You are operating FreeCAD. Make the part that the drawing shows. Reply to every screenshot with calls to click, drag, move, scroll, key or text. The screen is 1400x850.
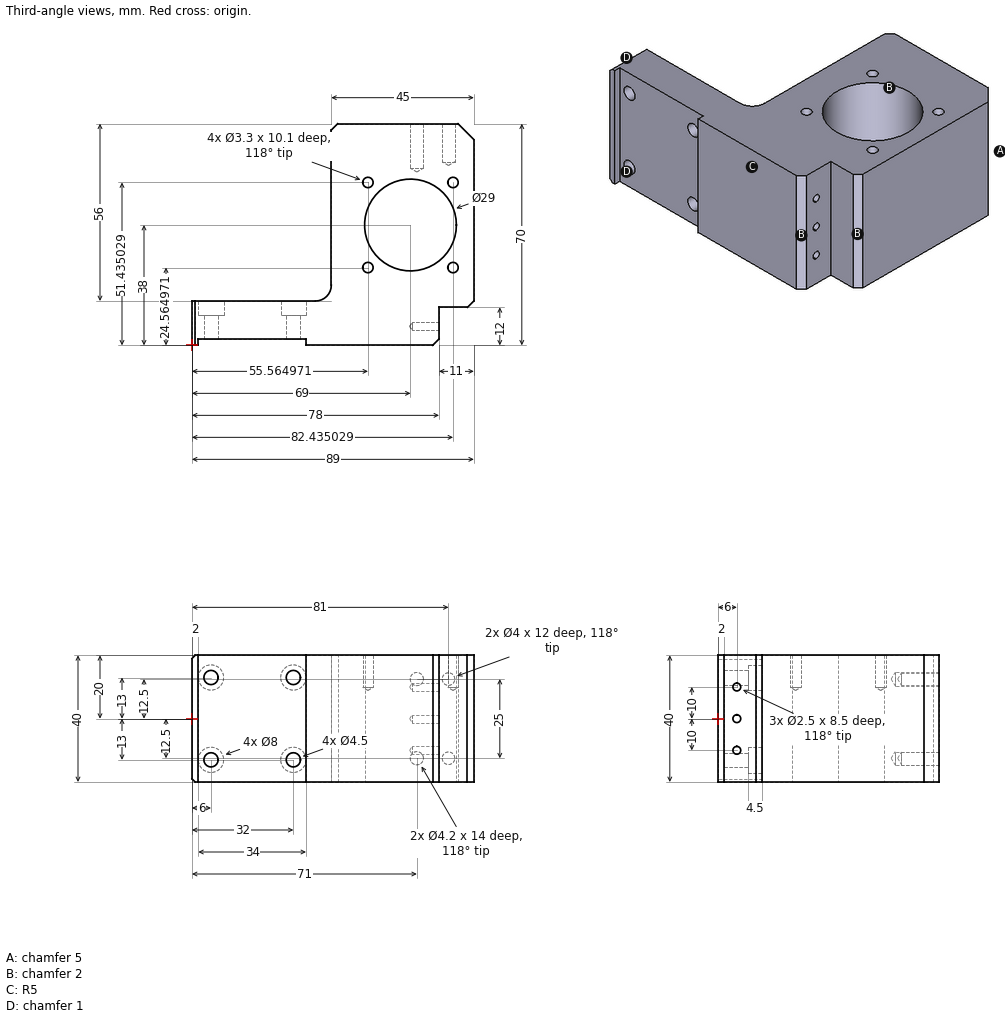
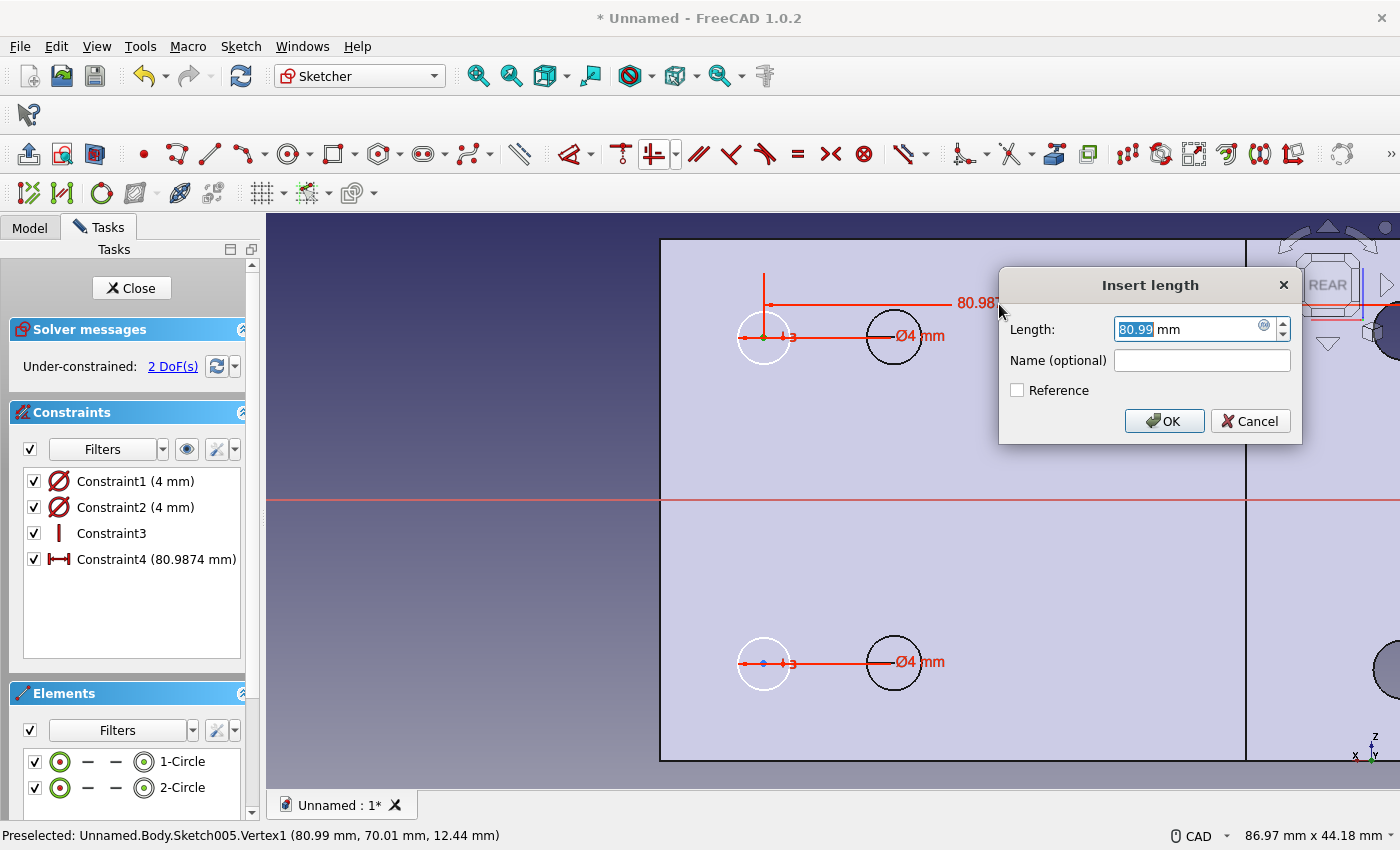
text(81)
key(Return)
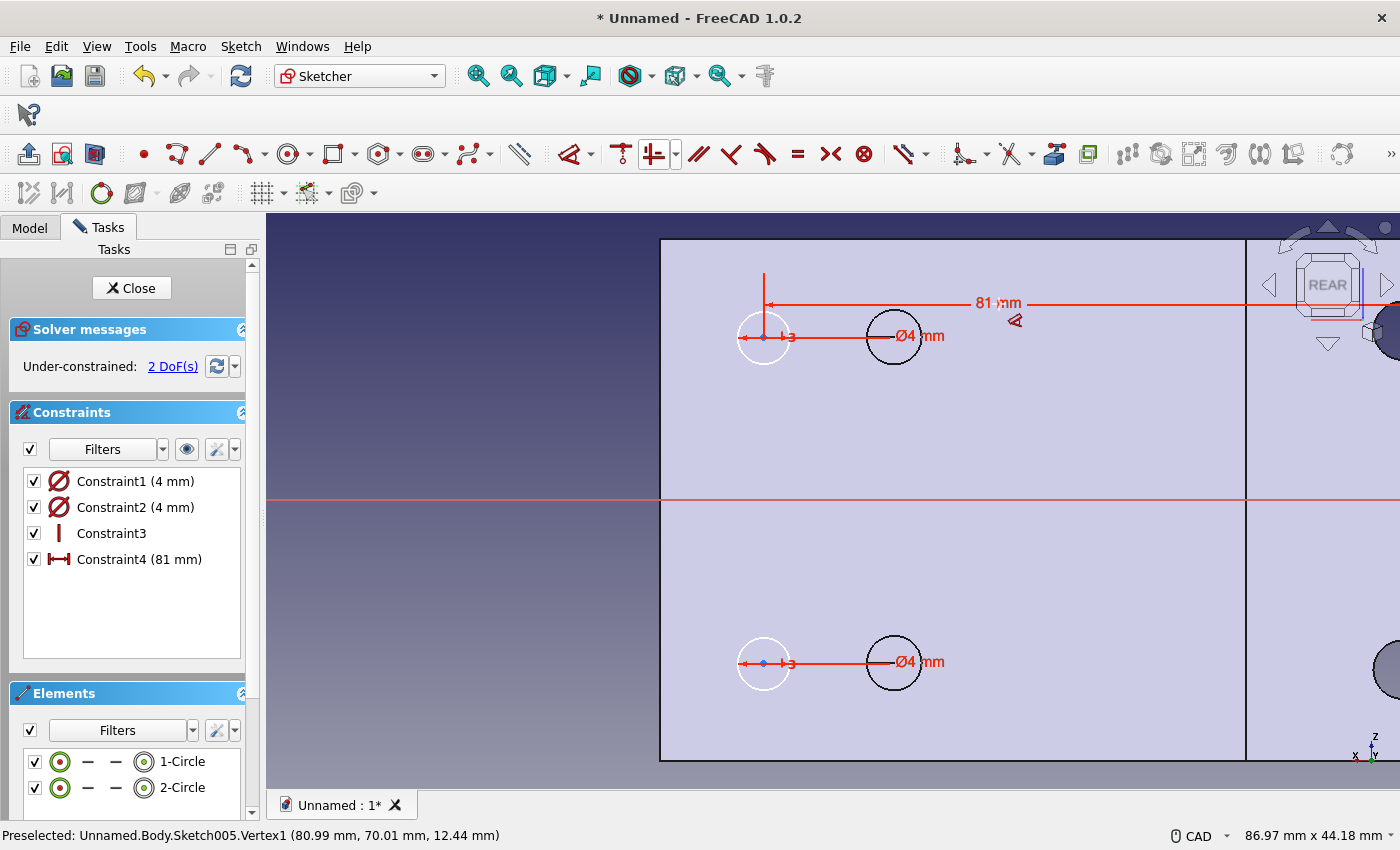
click(764, 338)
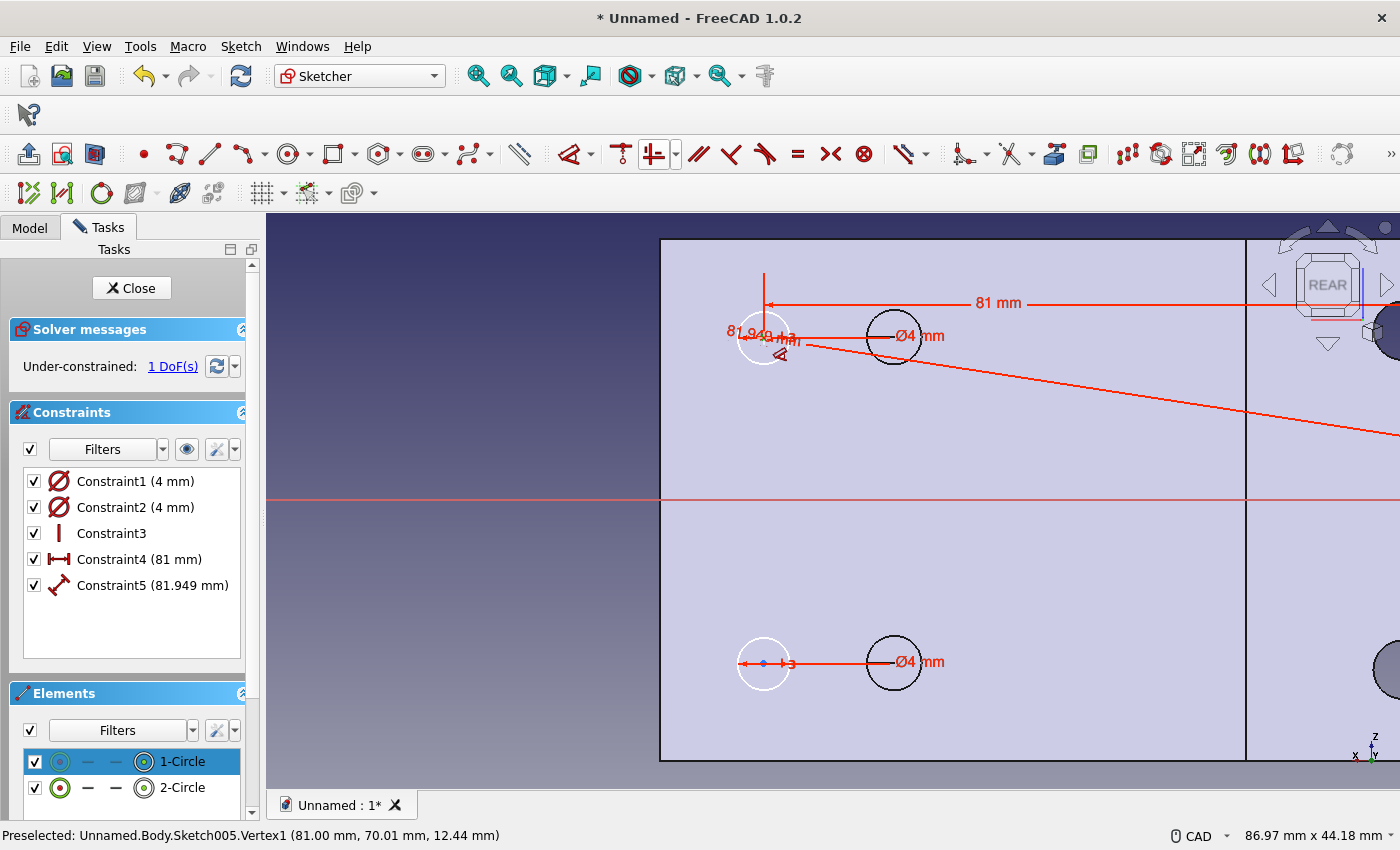
click(764, 664)
click(798, 426)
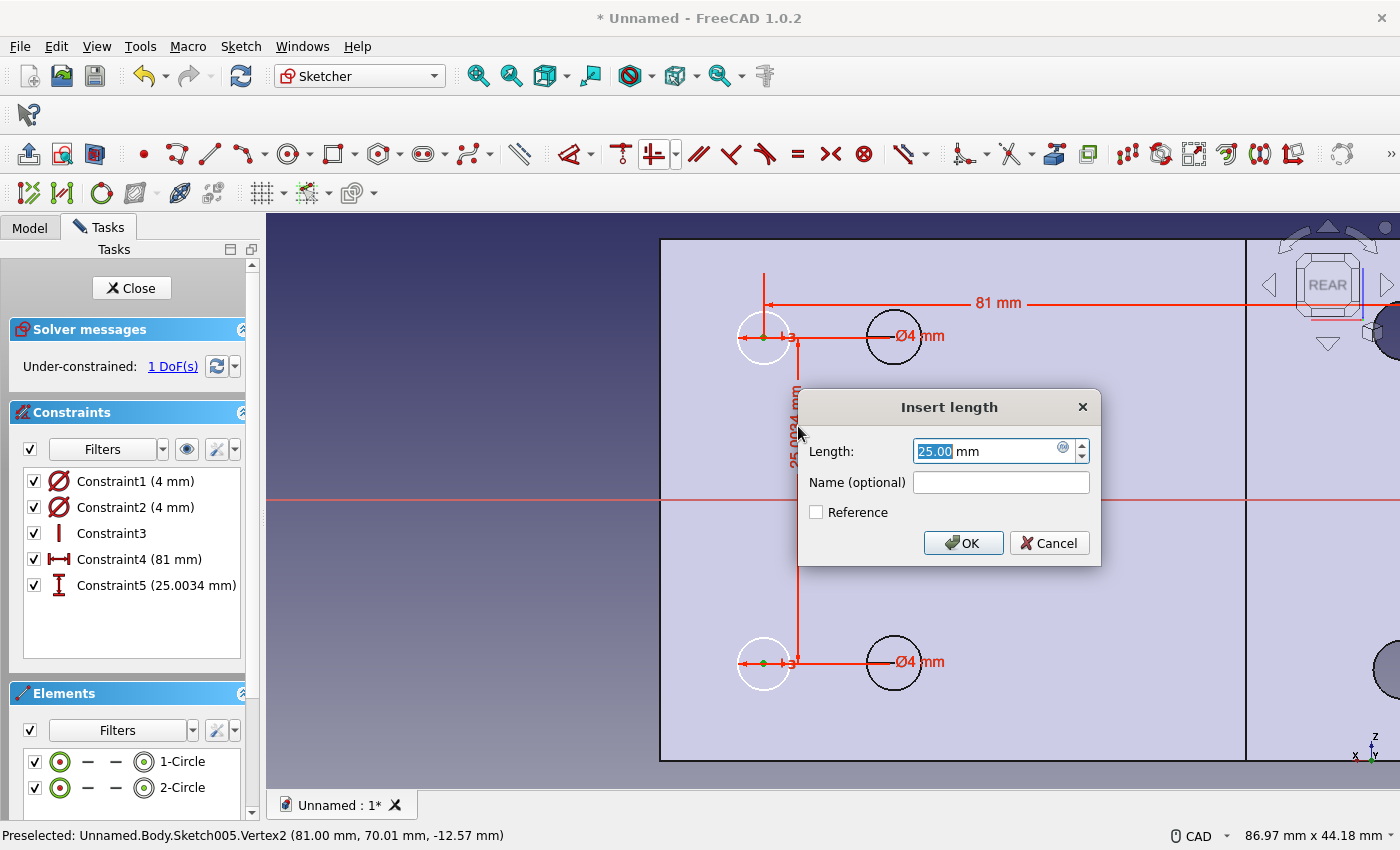
text(25)
key(Return)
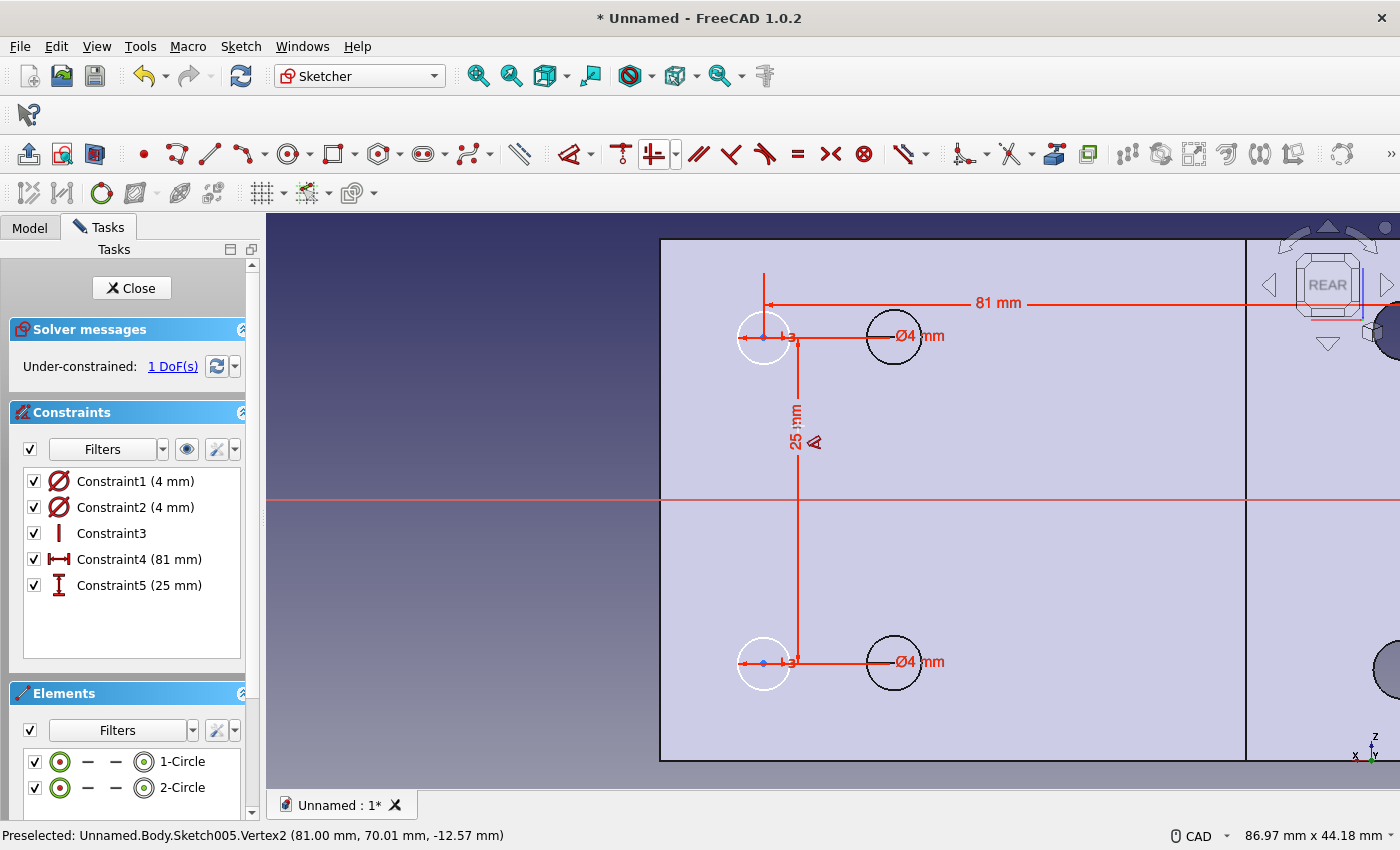
click(764, 338)
click(730, 382)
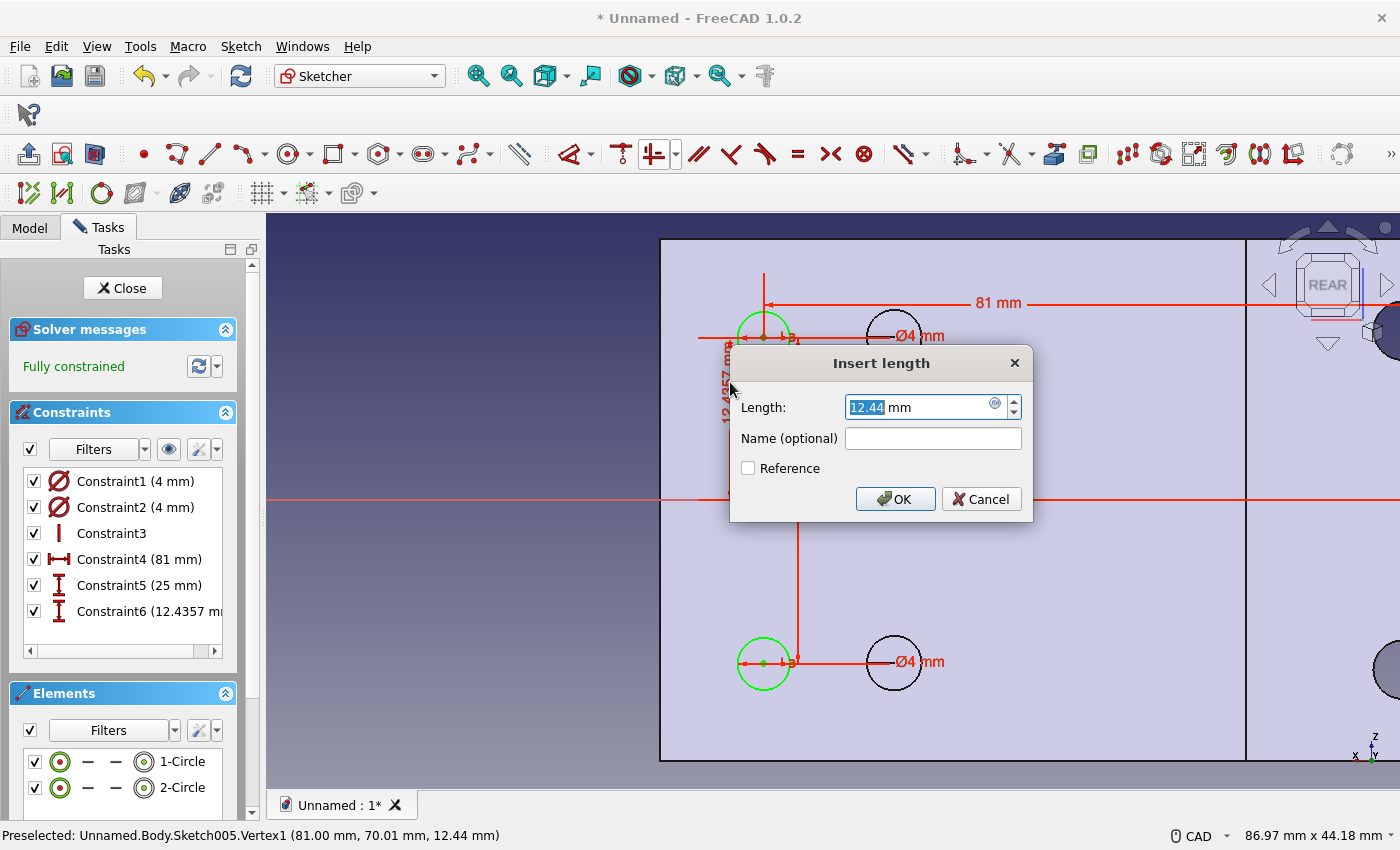
text(12.5)
key(Return)
key(Escape)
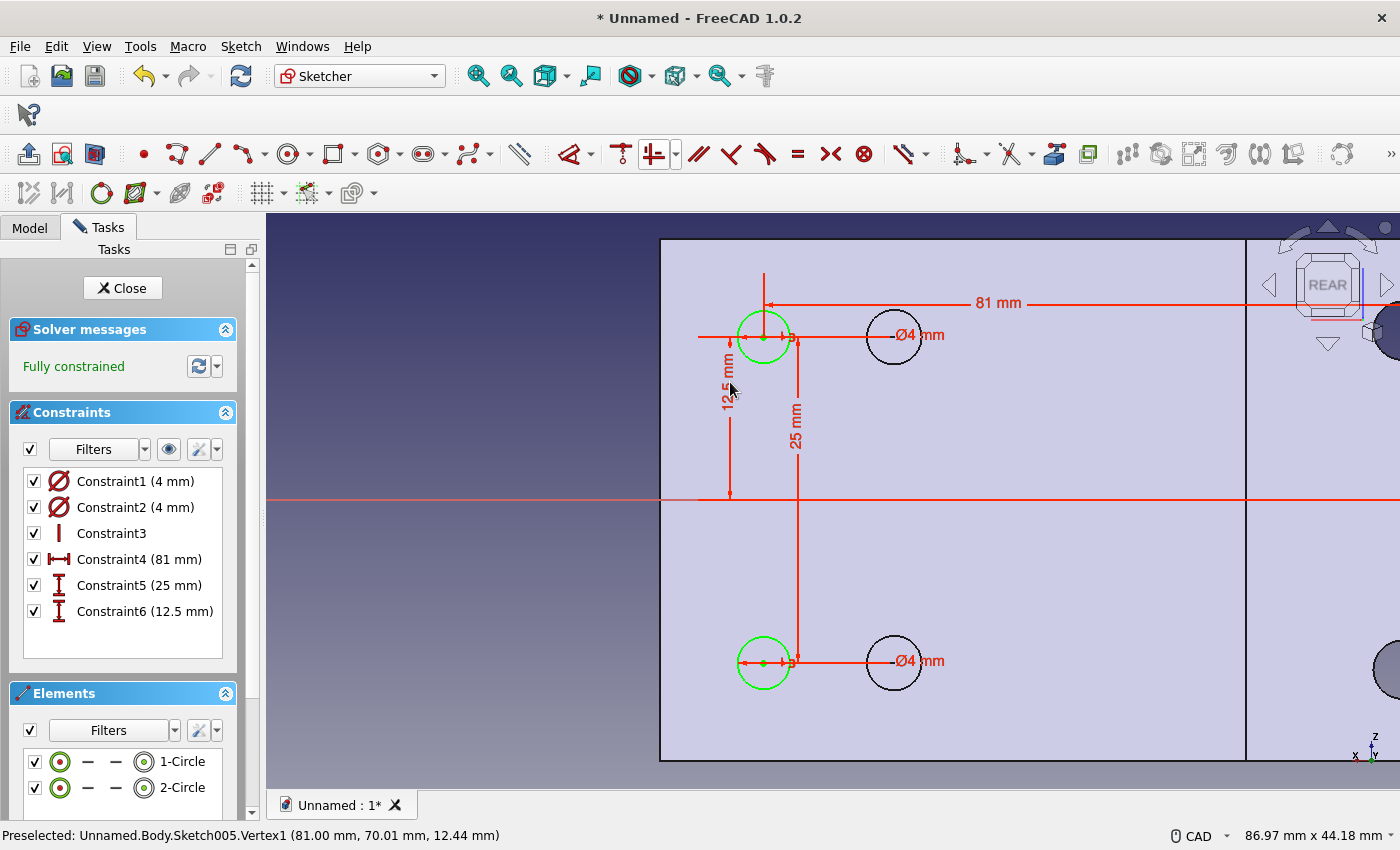
click(123, 288)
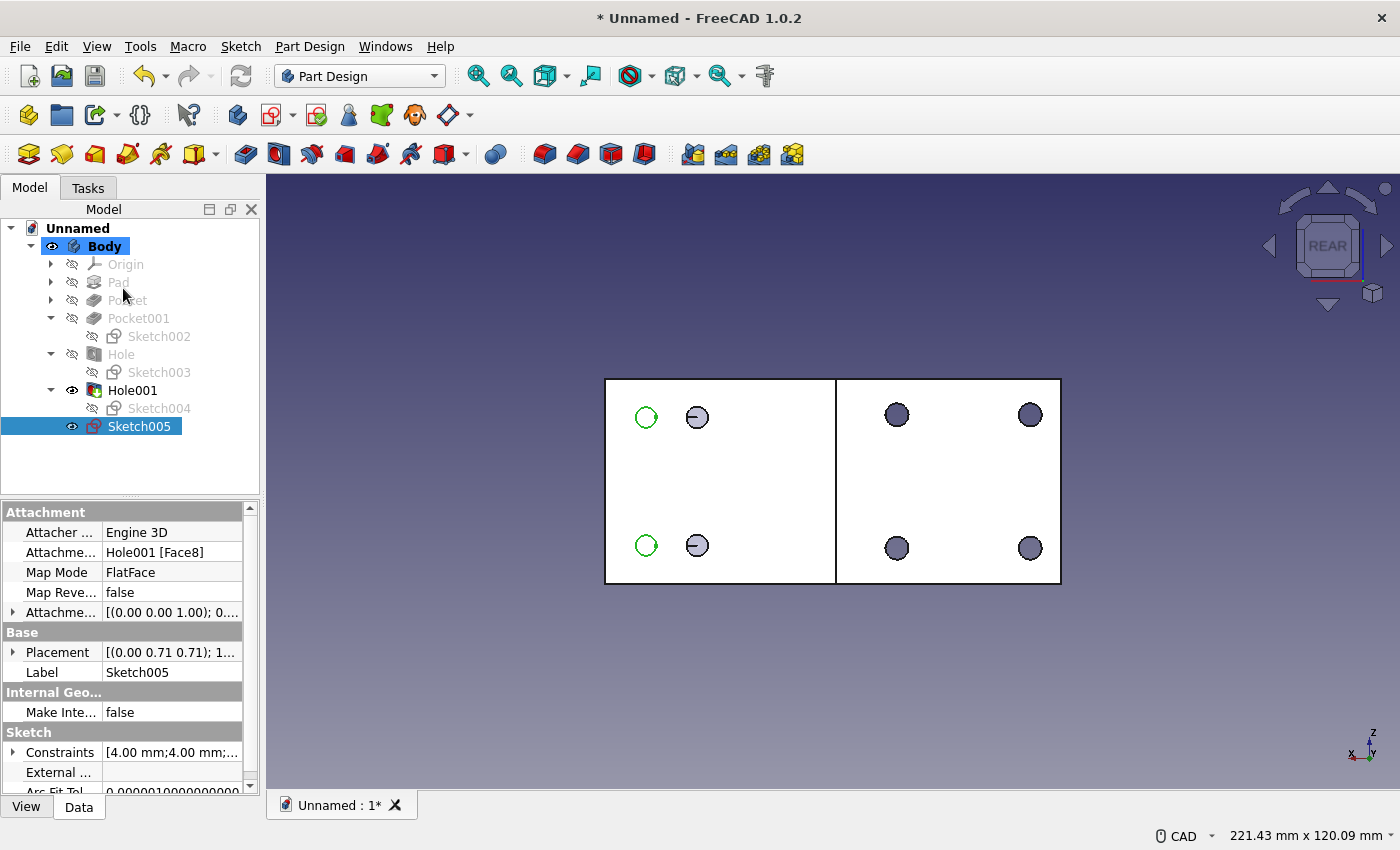
click(279, 154)